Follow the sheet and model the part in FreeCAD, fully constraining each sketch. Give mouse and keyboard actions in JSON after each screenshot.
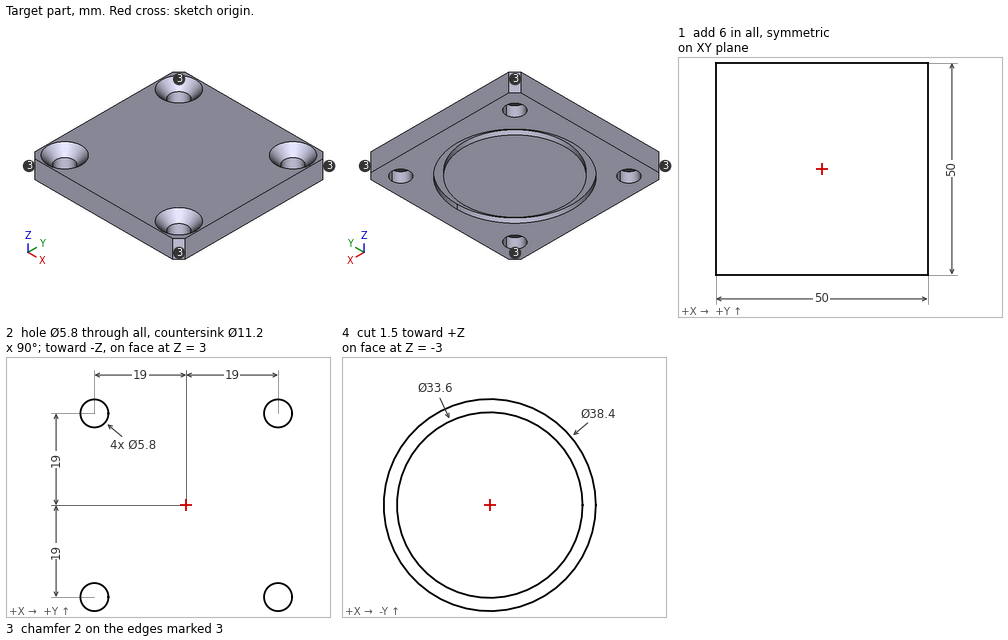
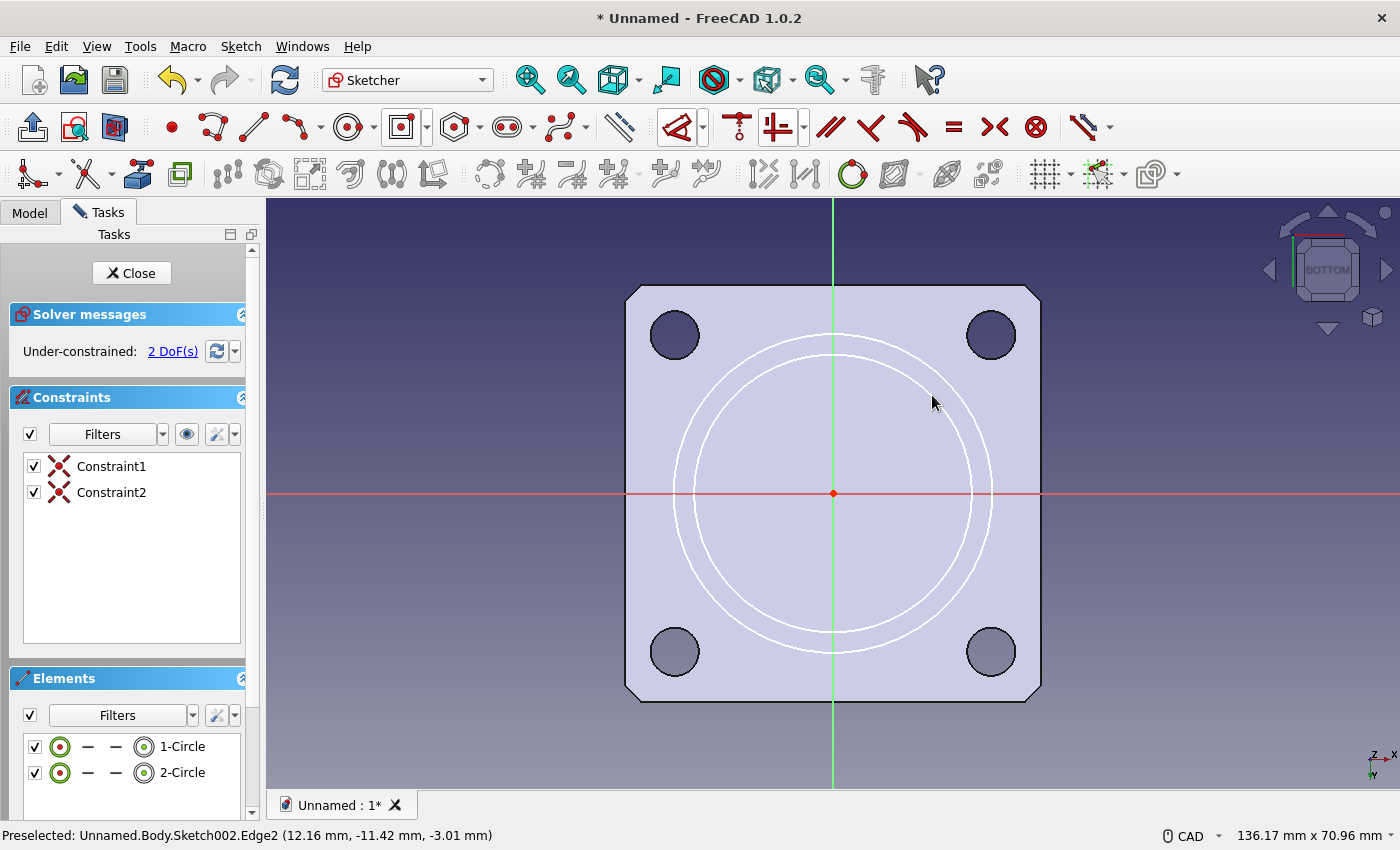
{"action": "left_click", "coordinate": [945, 380]}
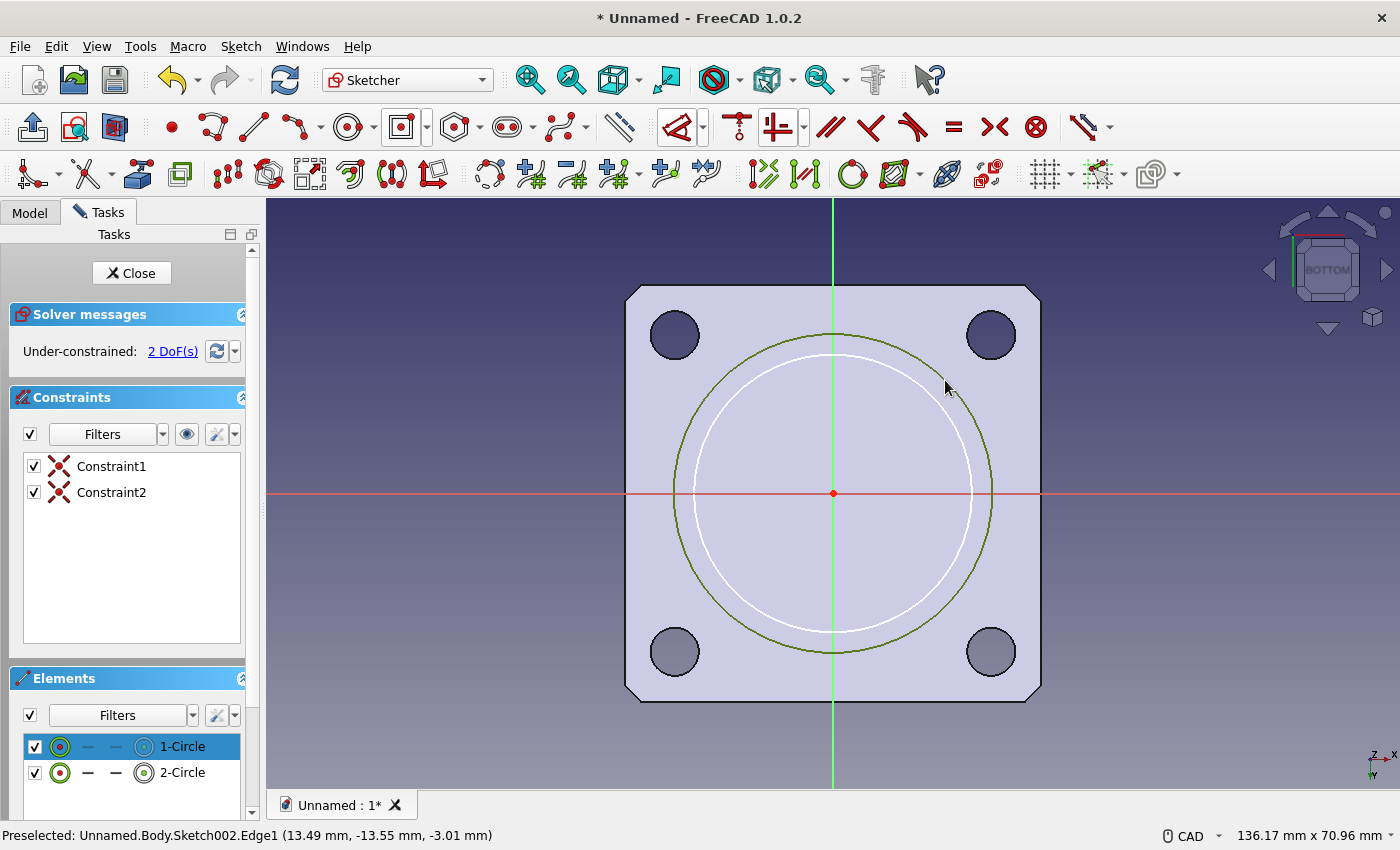
{"action": "key", "text": "k o"}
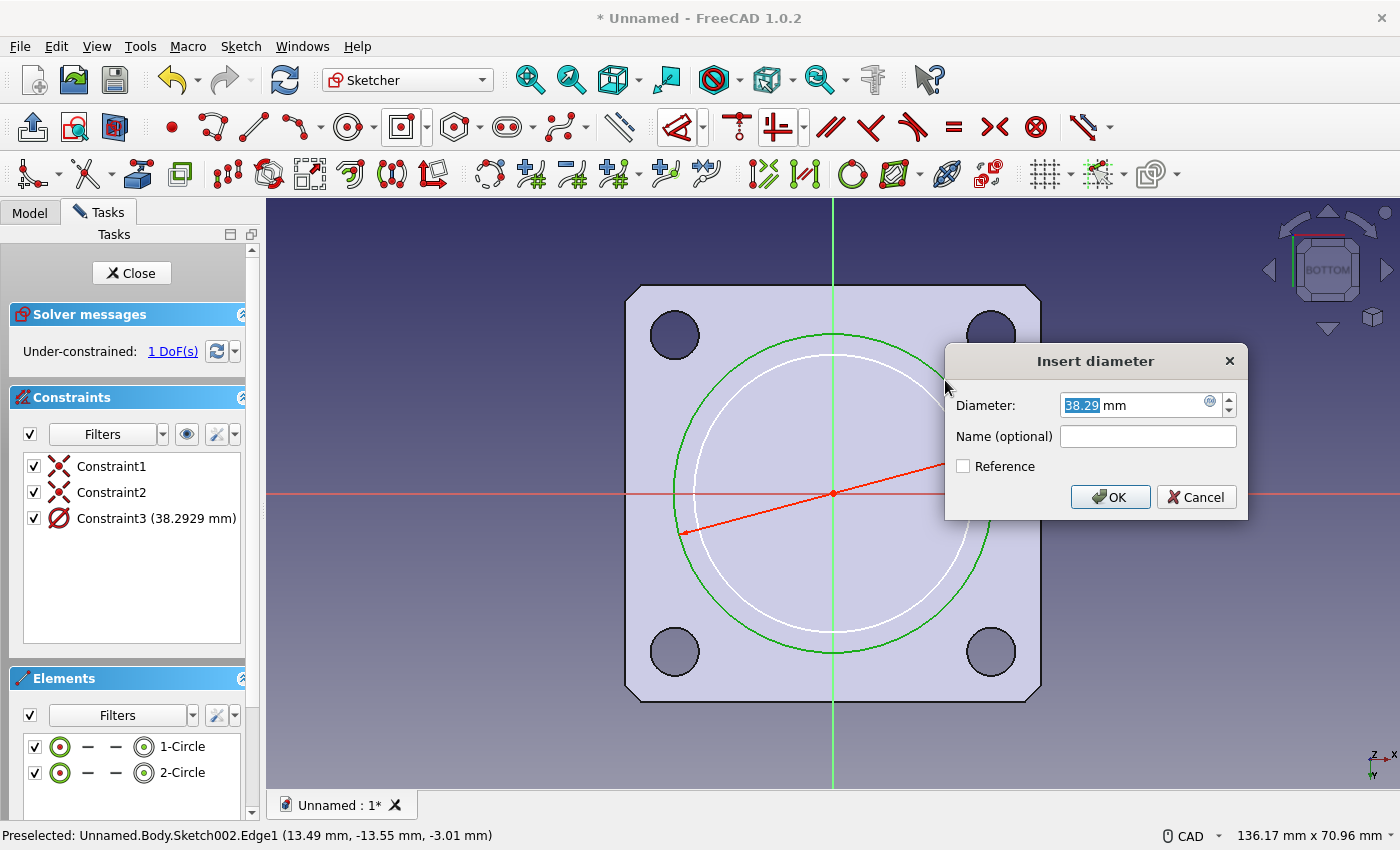
{"action": "type", "text": "38.4"}
{"action": "key", "text": "Return"}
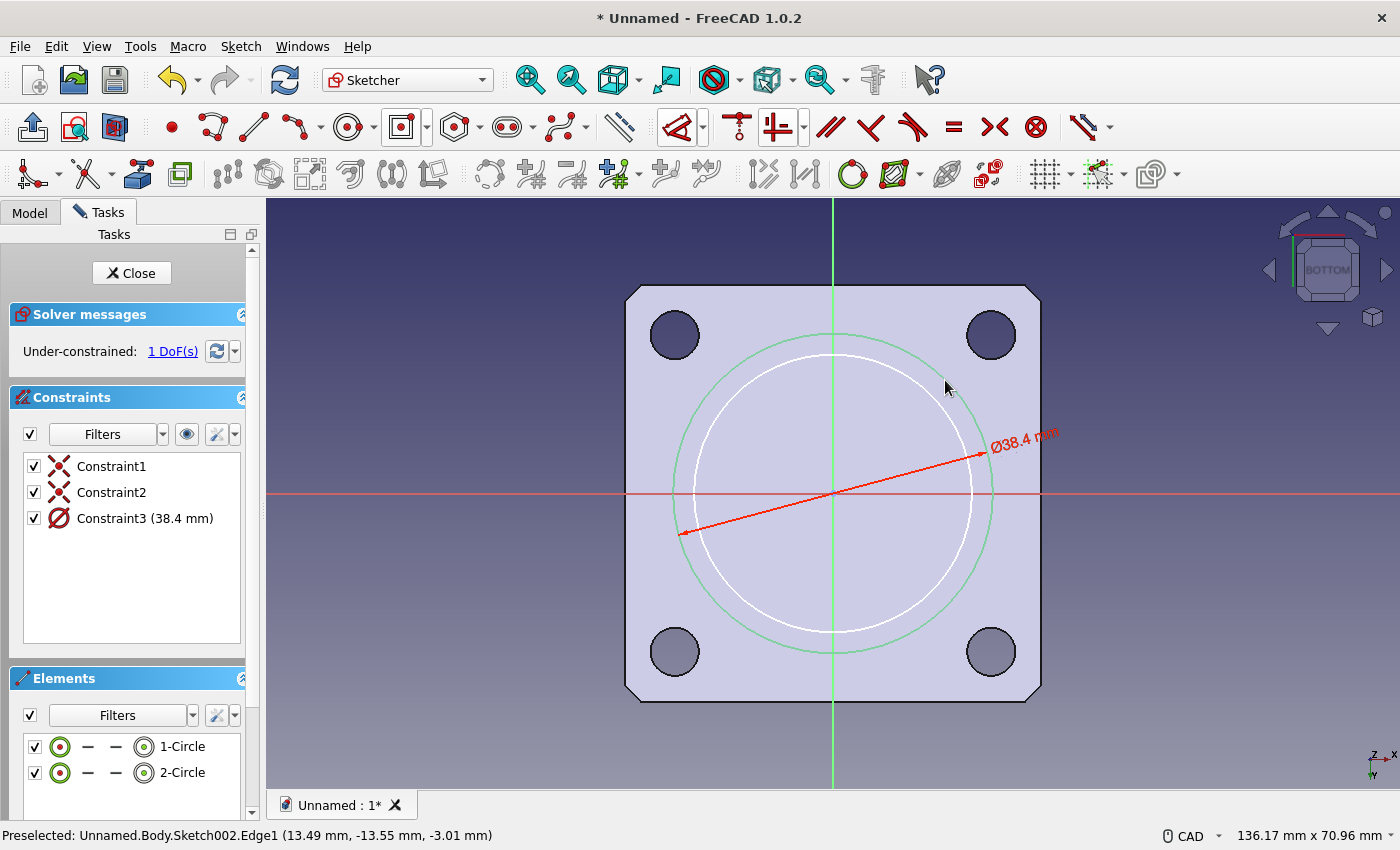
{"action": "left_click", "coordinate": [931, 395]}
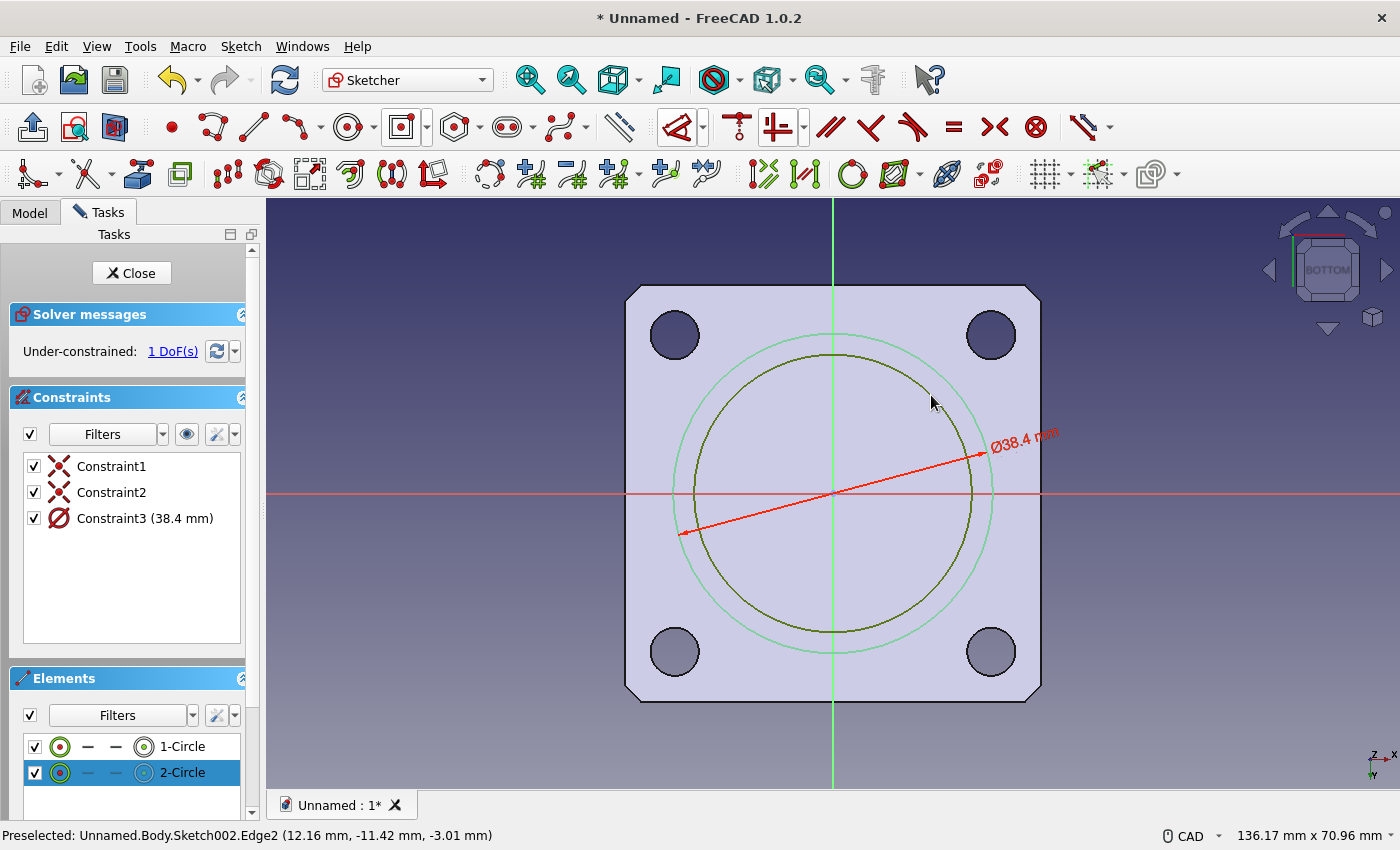
{"action": "key", "text": "k o"}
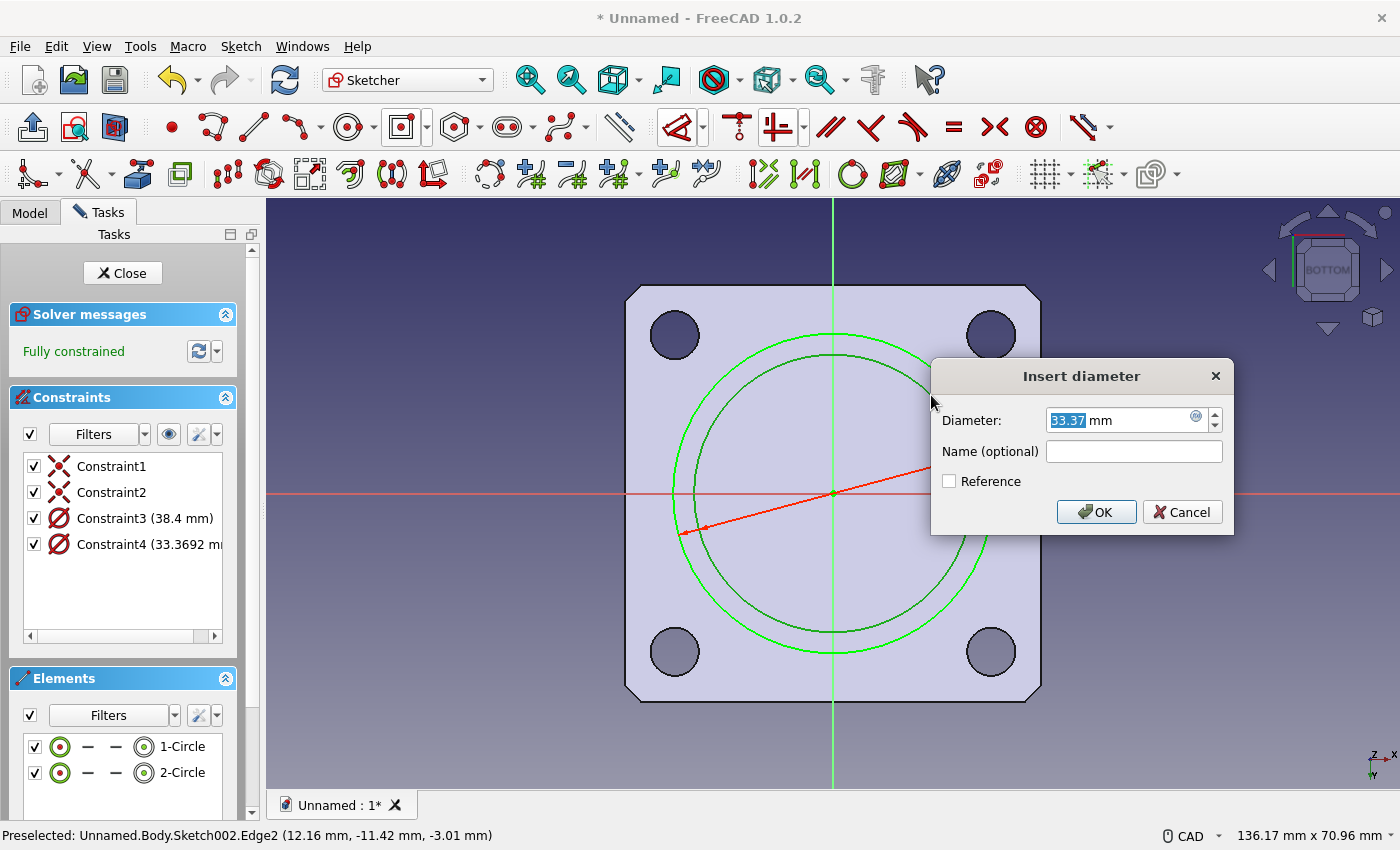
{"action": "type", "text": "33.6"}
{"action": "key", "text": "Return"}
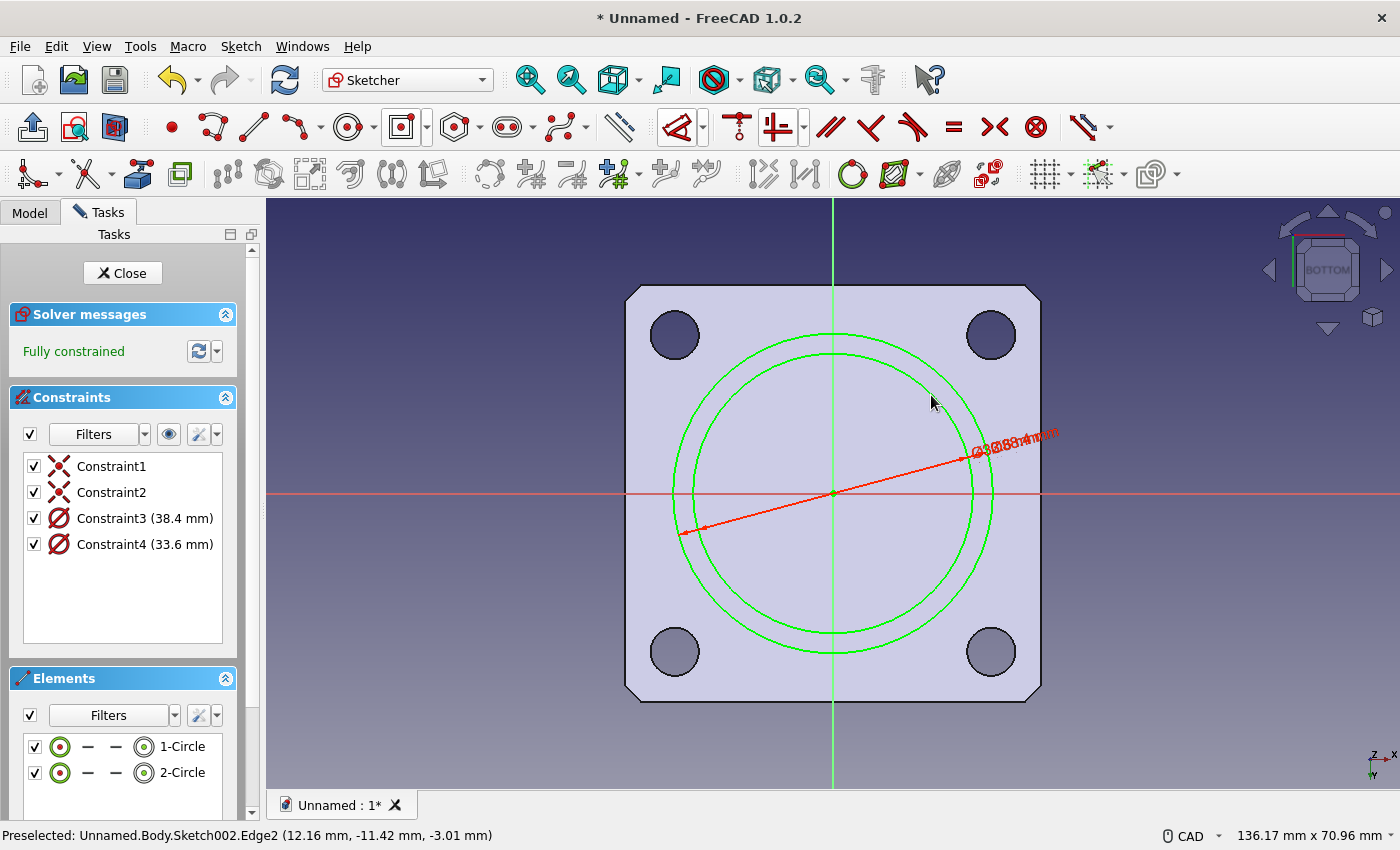
{"action": "left_click", "coordinate": [123, 273]}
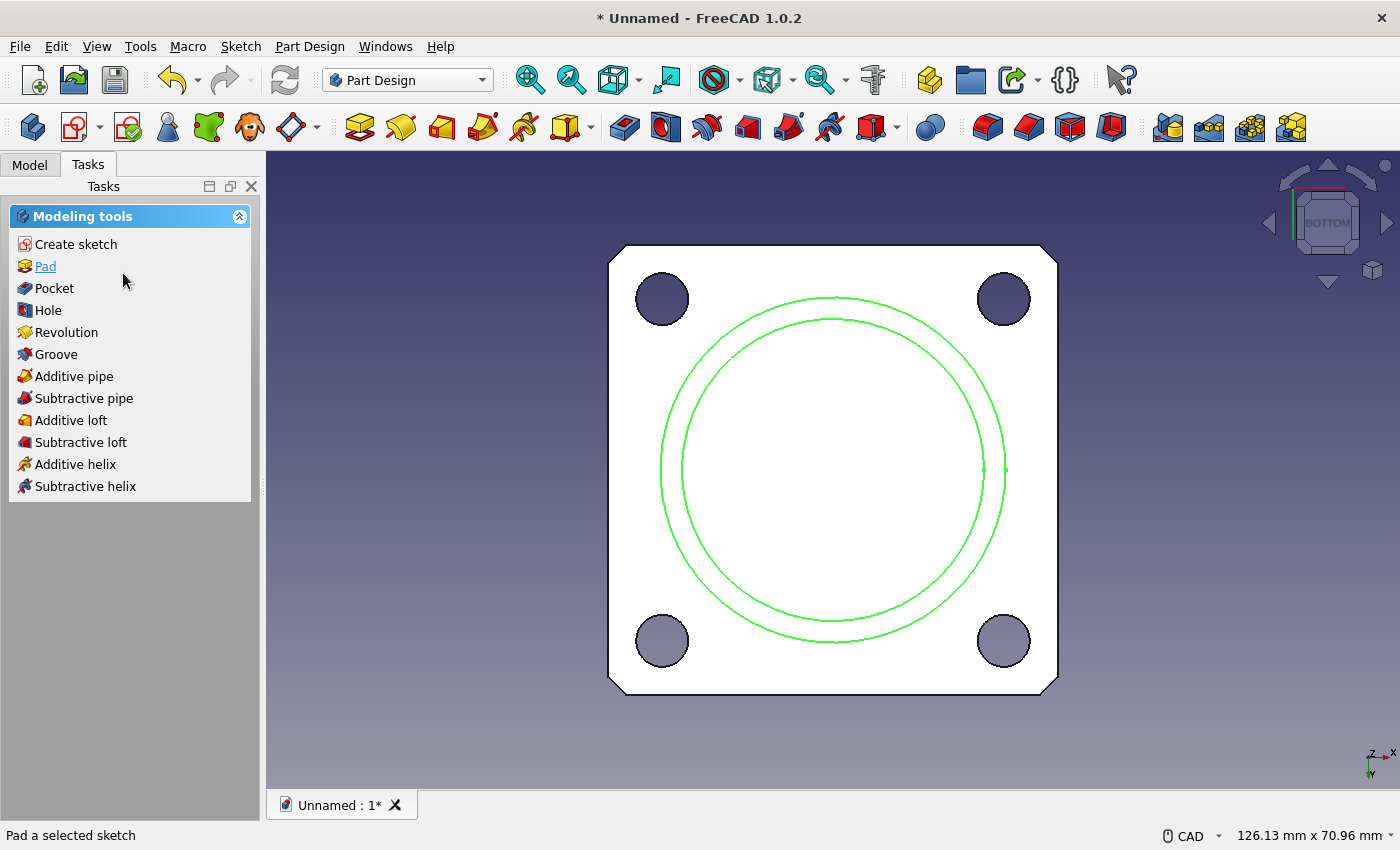
{"action": "left_click", "coordinate": [625, 128]}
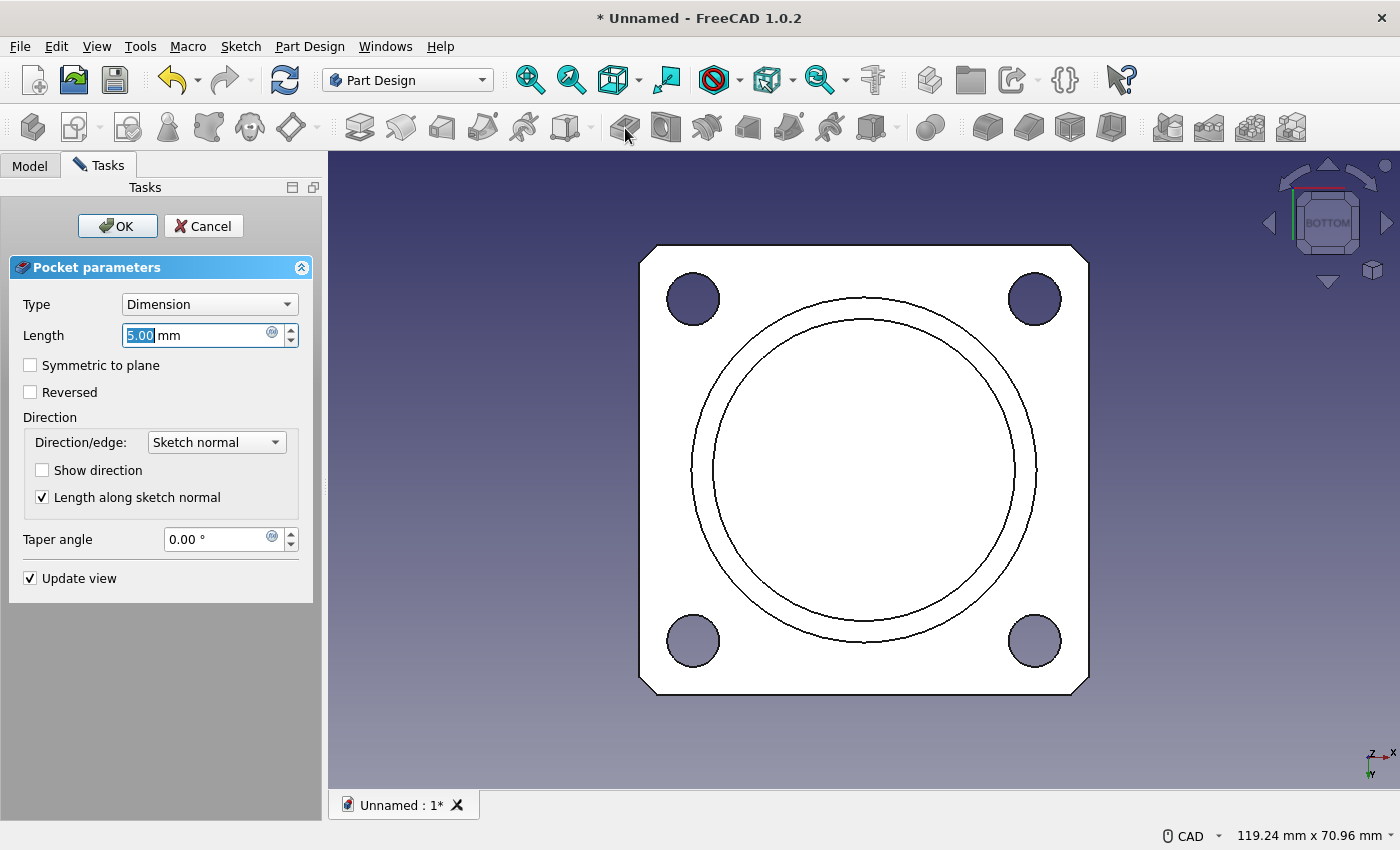
{"action": "type", "text": "1.5"}
{"action": "key", "text": "Tab"}